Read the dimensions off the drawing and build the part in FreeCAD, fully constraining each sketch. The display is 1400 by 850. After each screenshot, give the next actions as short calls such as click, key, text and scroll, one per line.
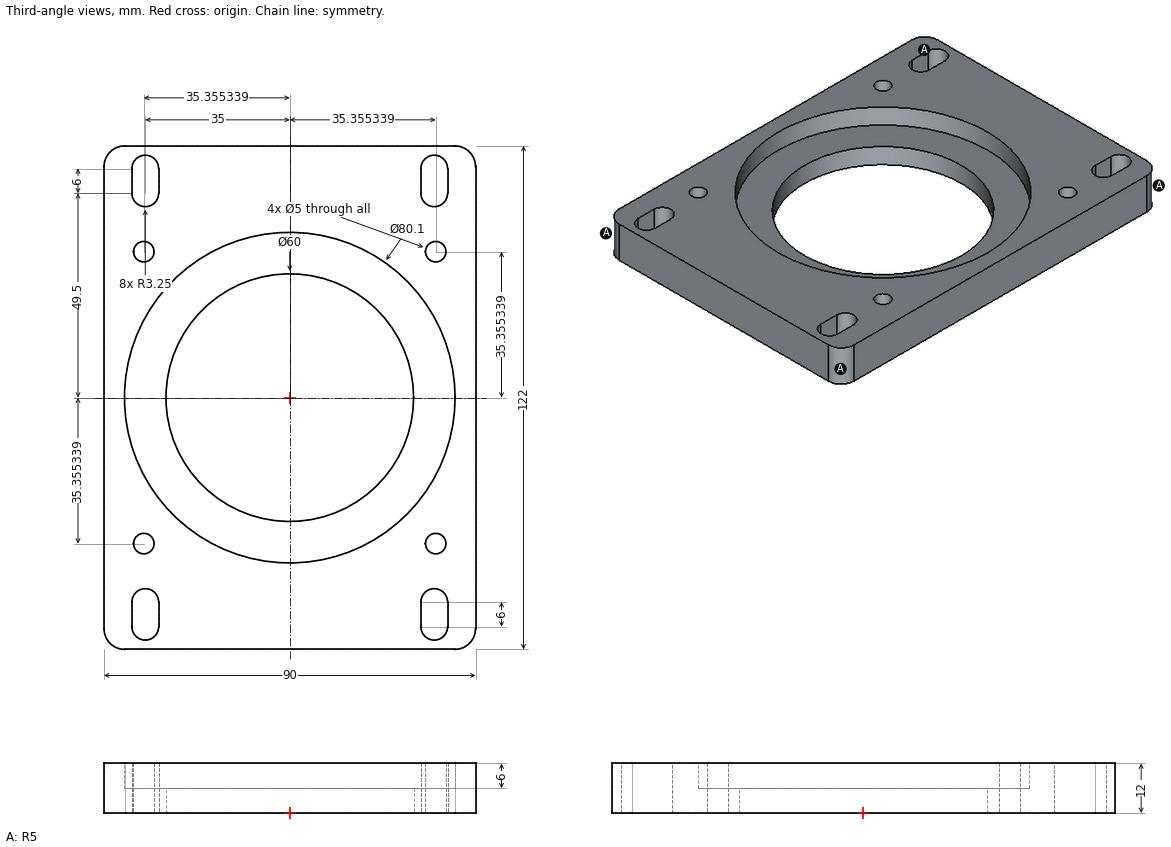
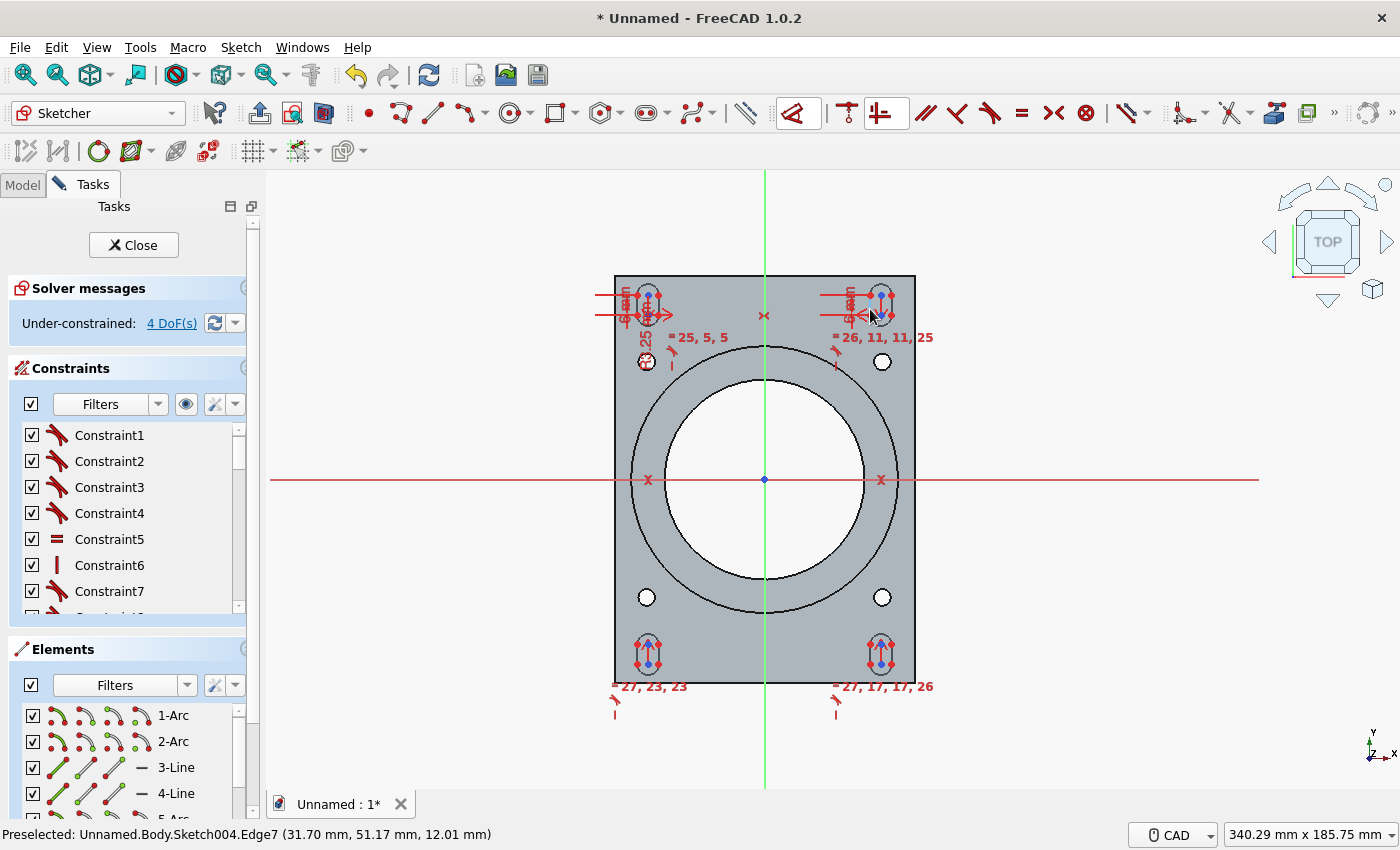
scroll(870, 658, up, 5)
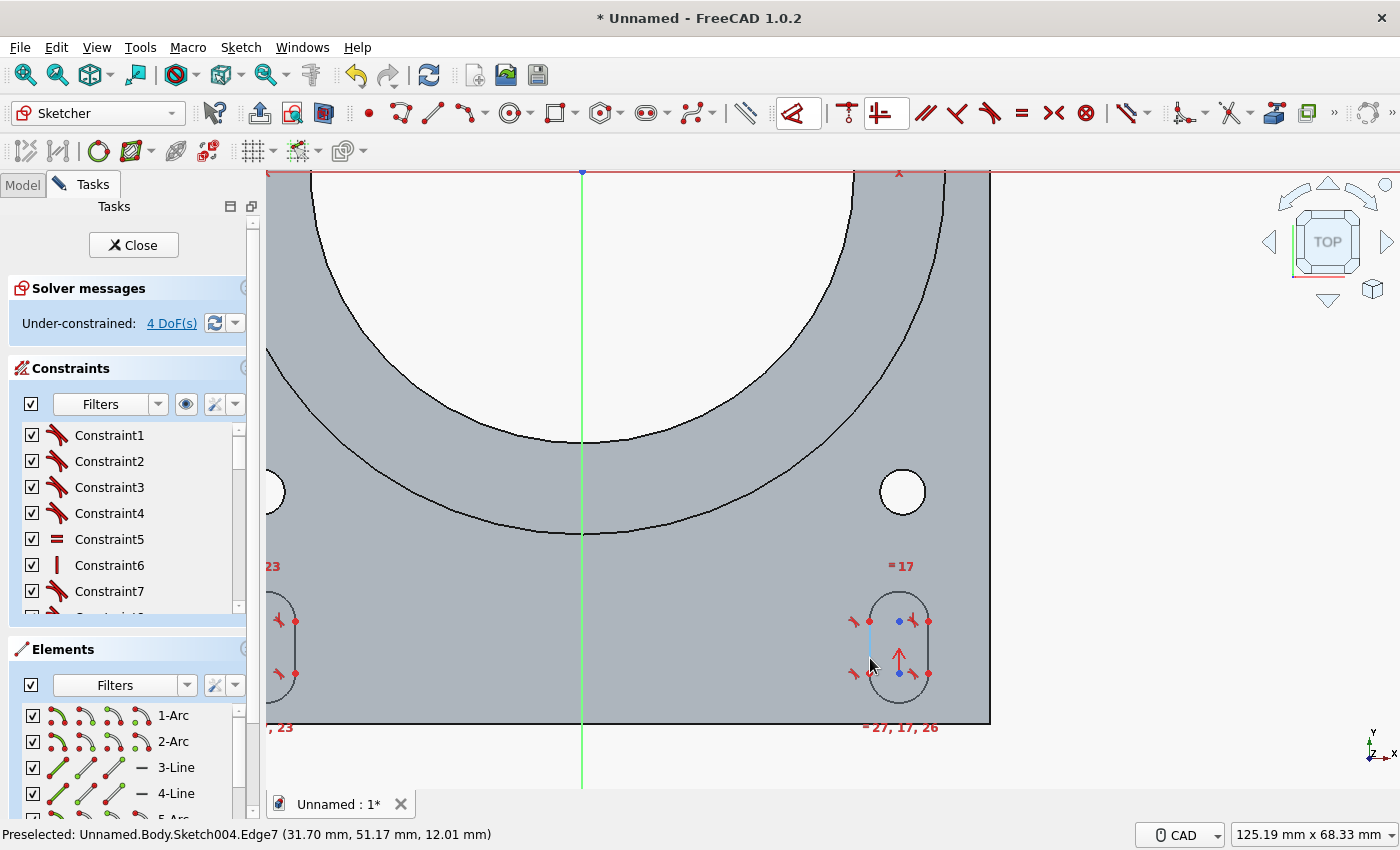
click(870, 658)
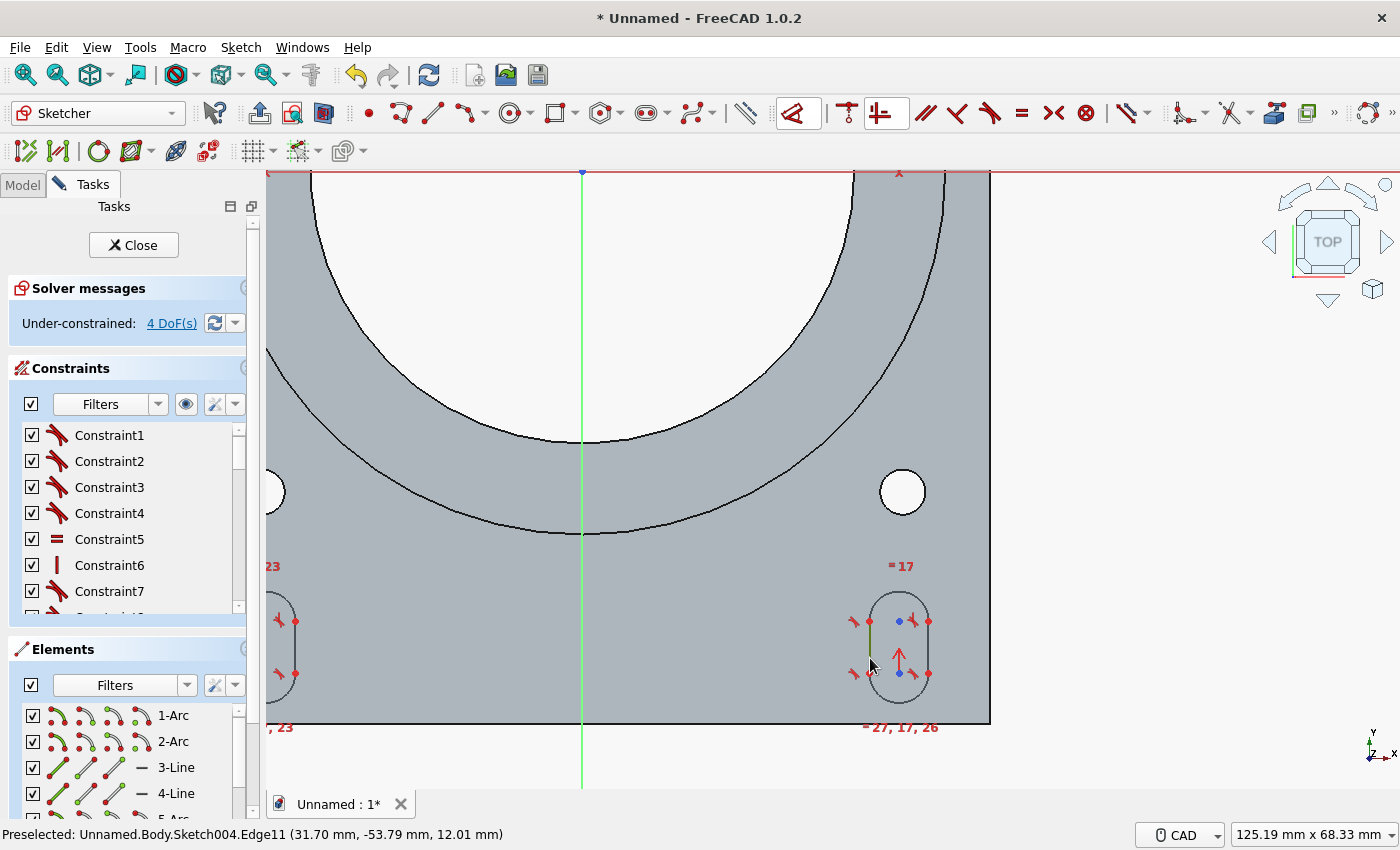
click(816, 114)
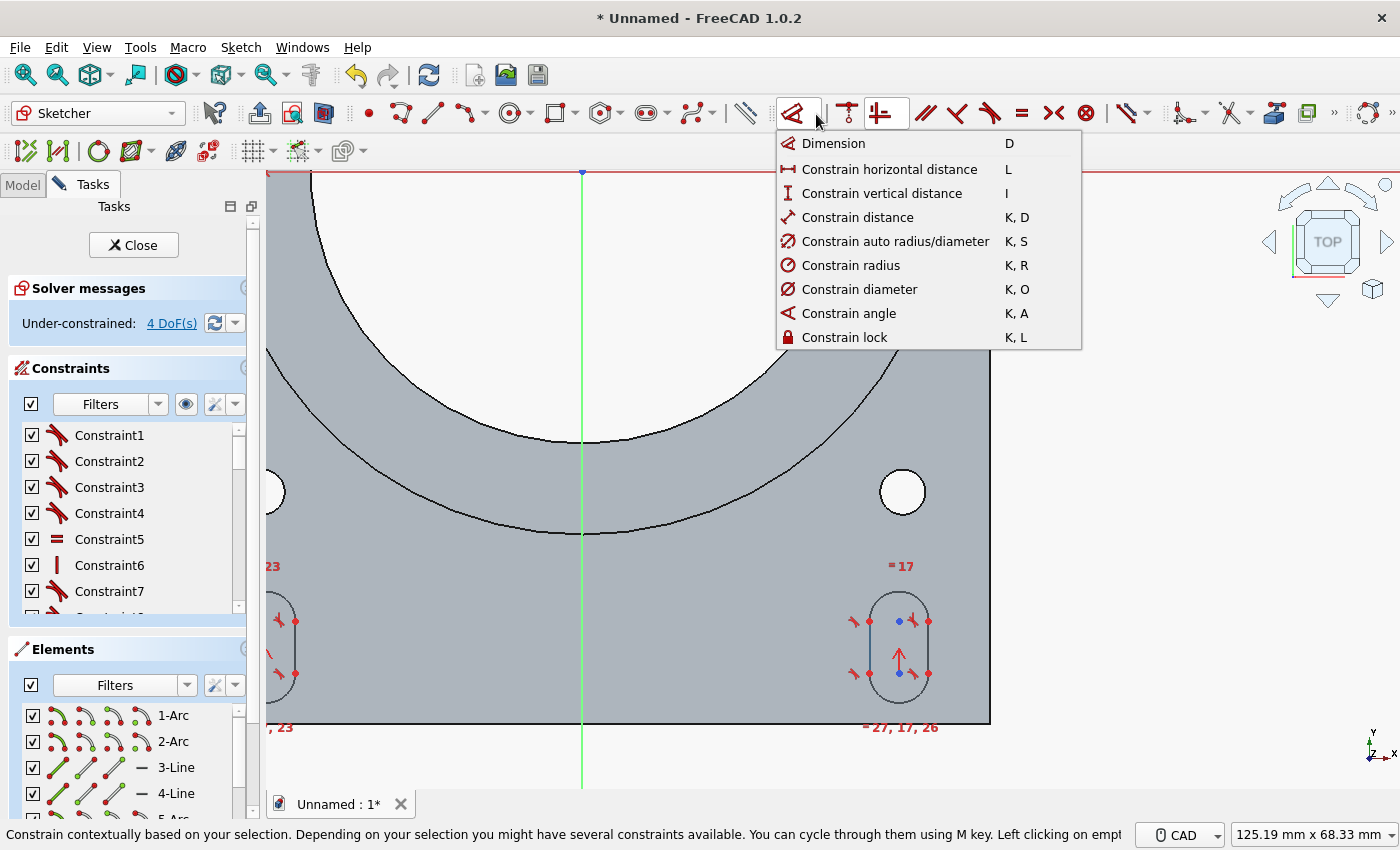
click(929, 193)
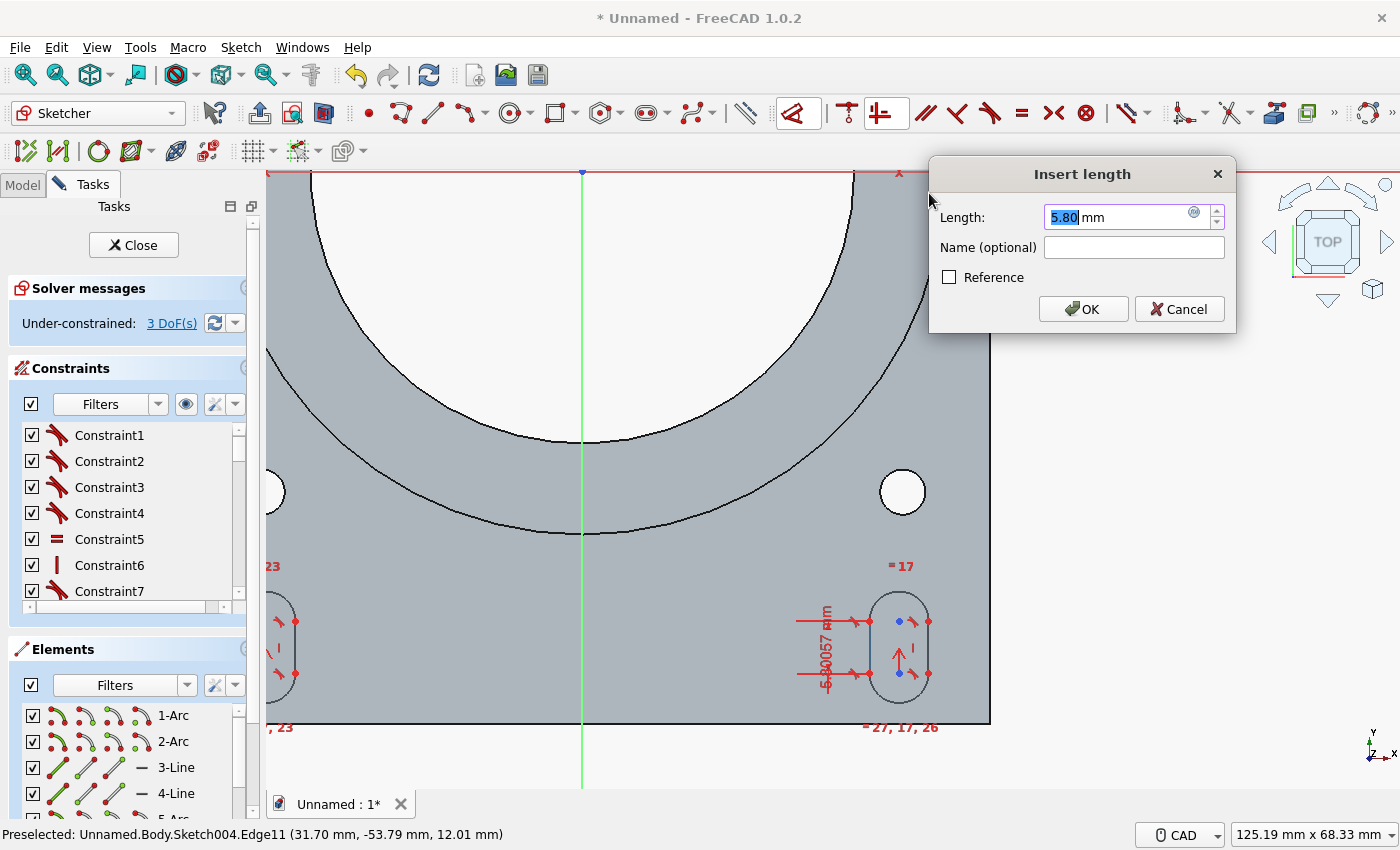
text(6)
key(Return)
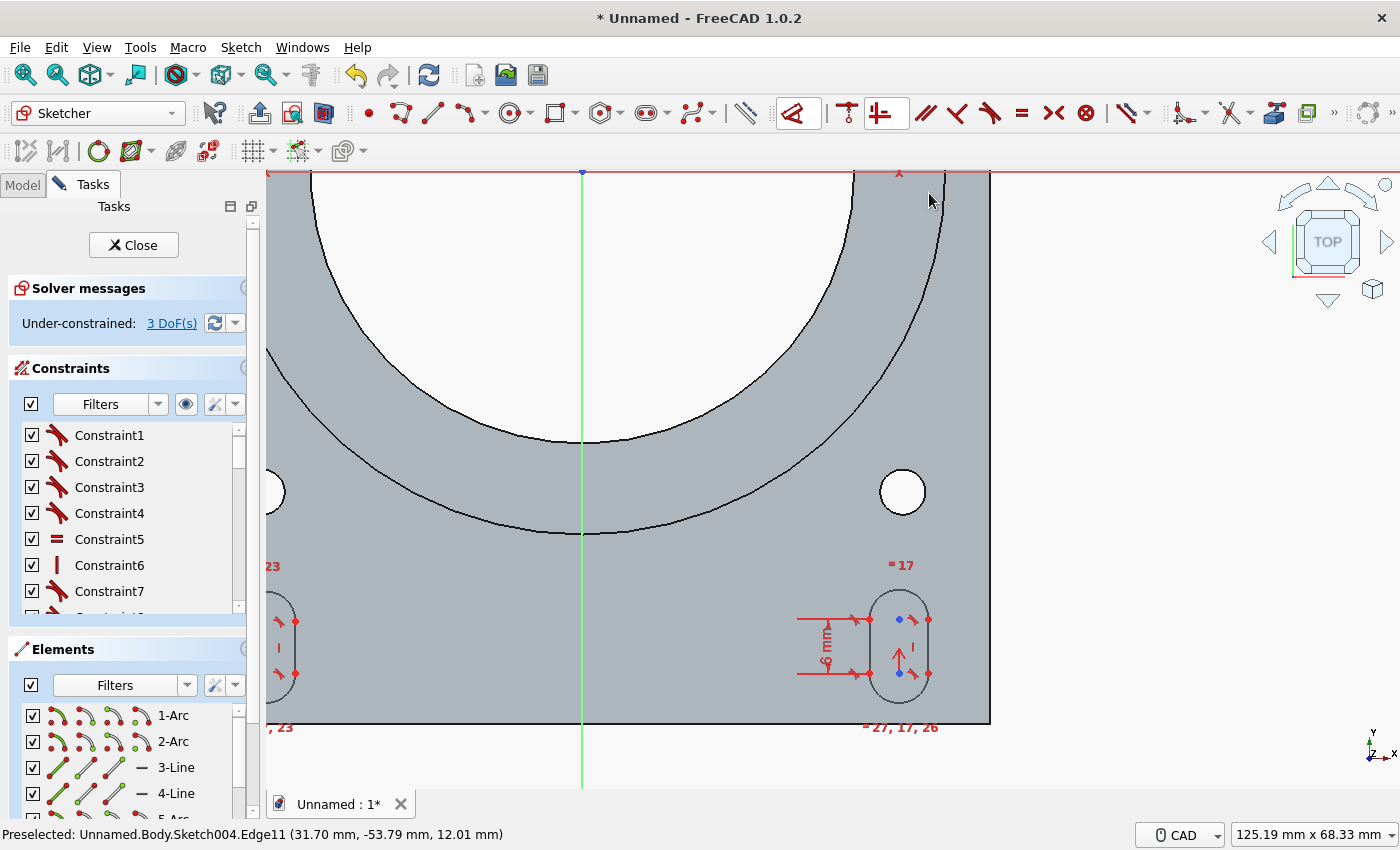
scroll(870, 659, down, 5)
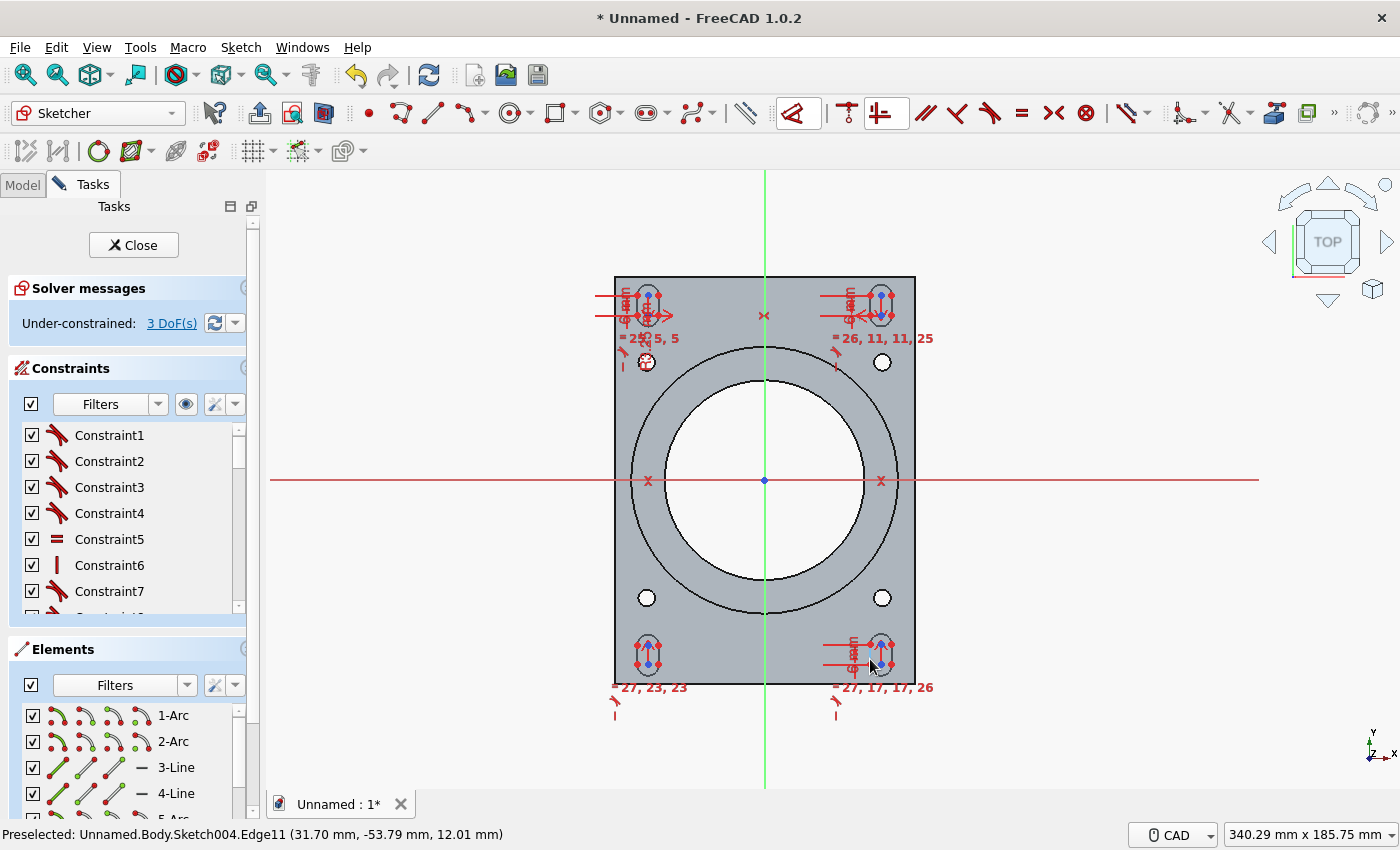
scroll(637, 659, up, 5)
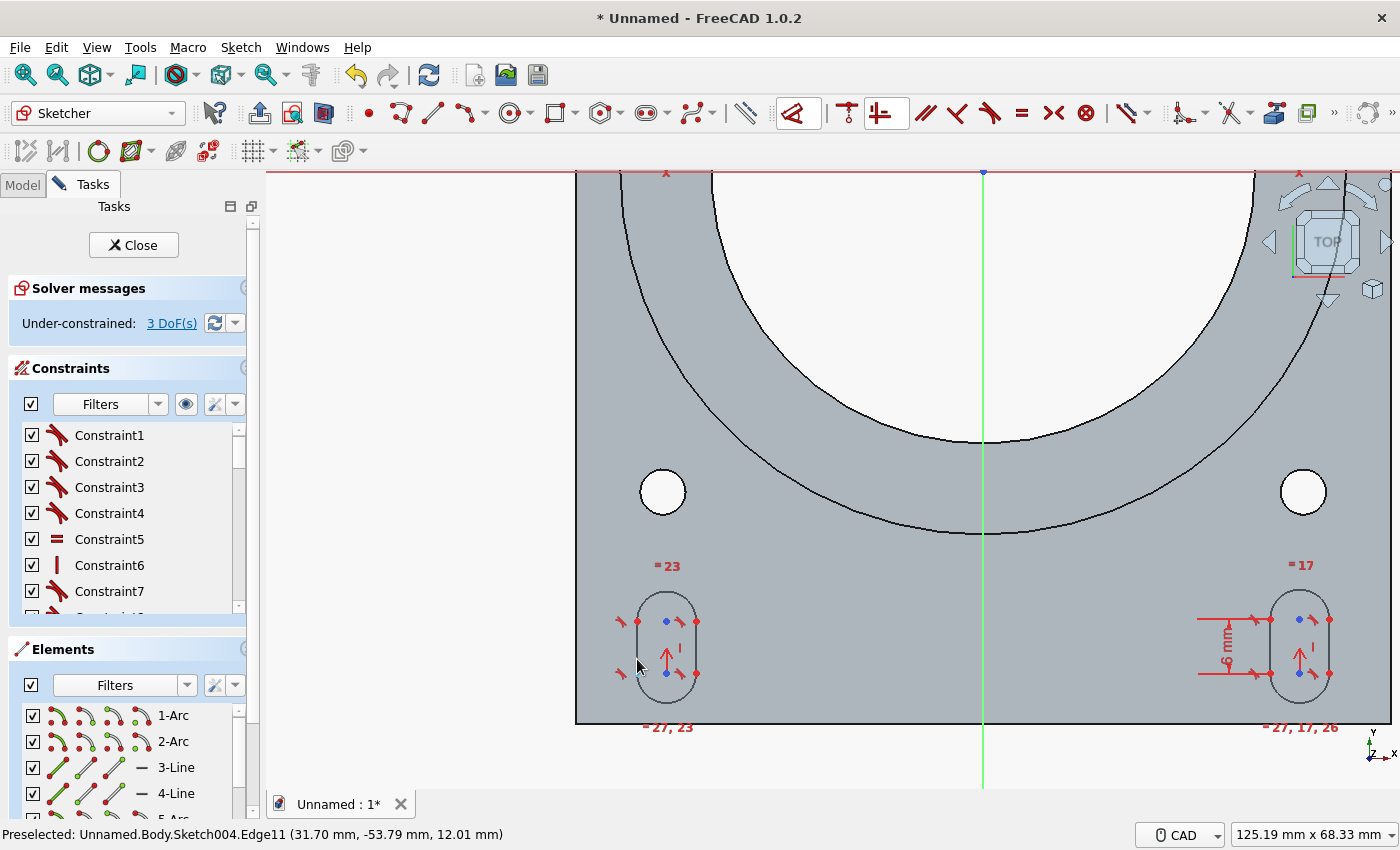
click(637, 658)